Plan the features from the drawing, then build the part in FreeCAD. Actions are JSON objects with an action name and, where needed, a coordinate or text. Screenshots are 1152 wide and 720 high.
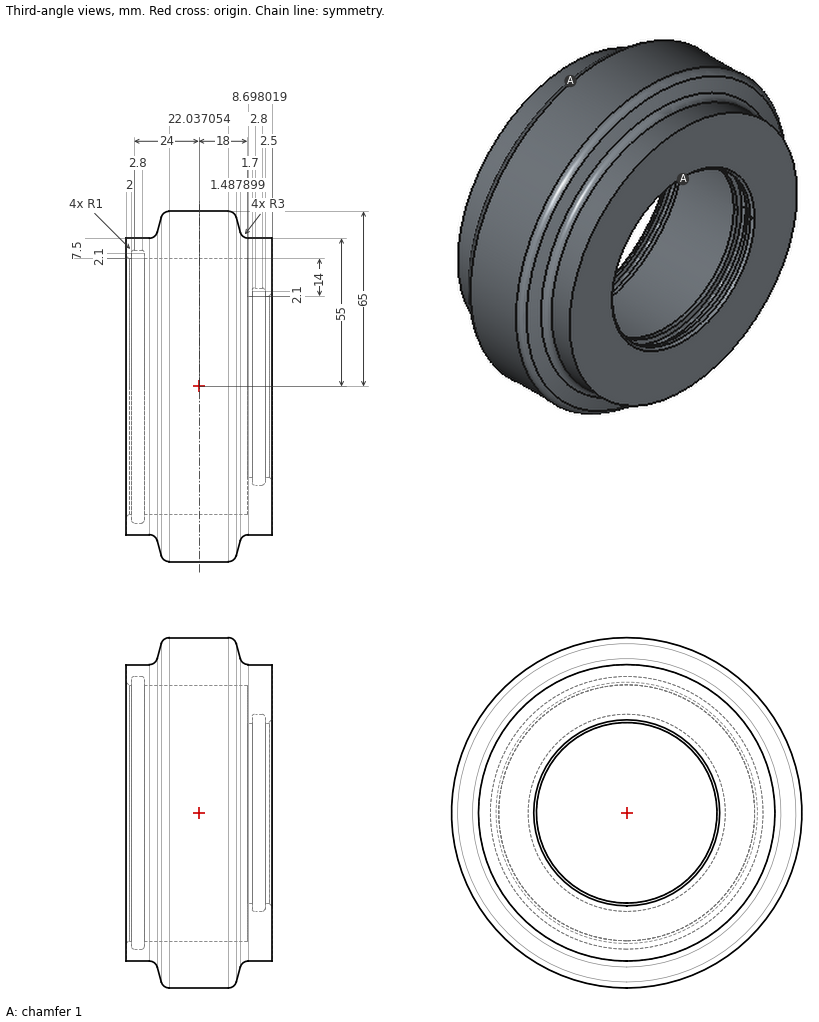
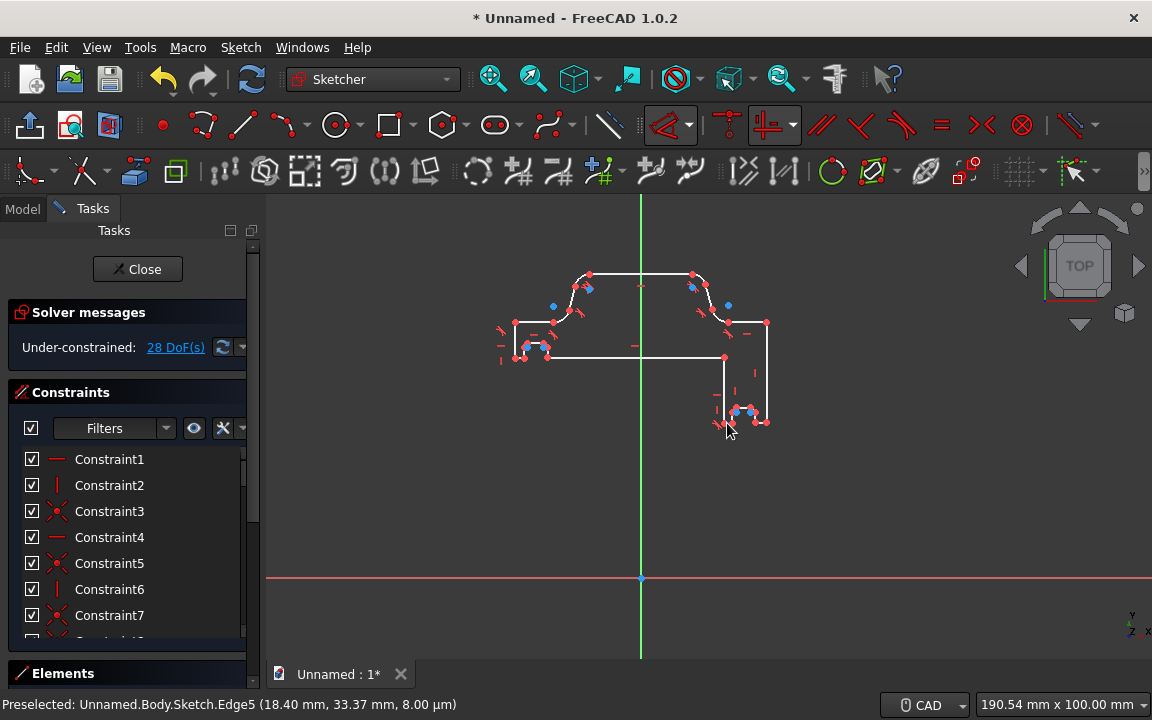
{"action": "scroll", "coordinate": [547, 346], "scroll_direction": "up", "scroll_amount": 10}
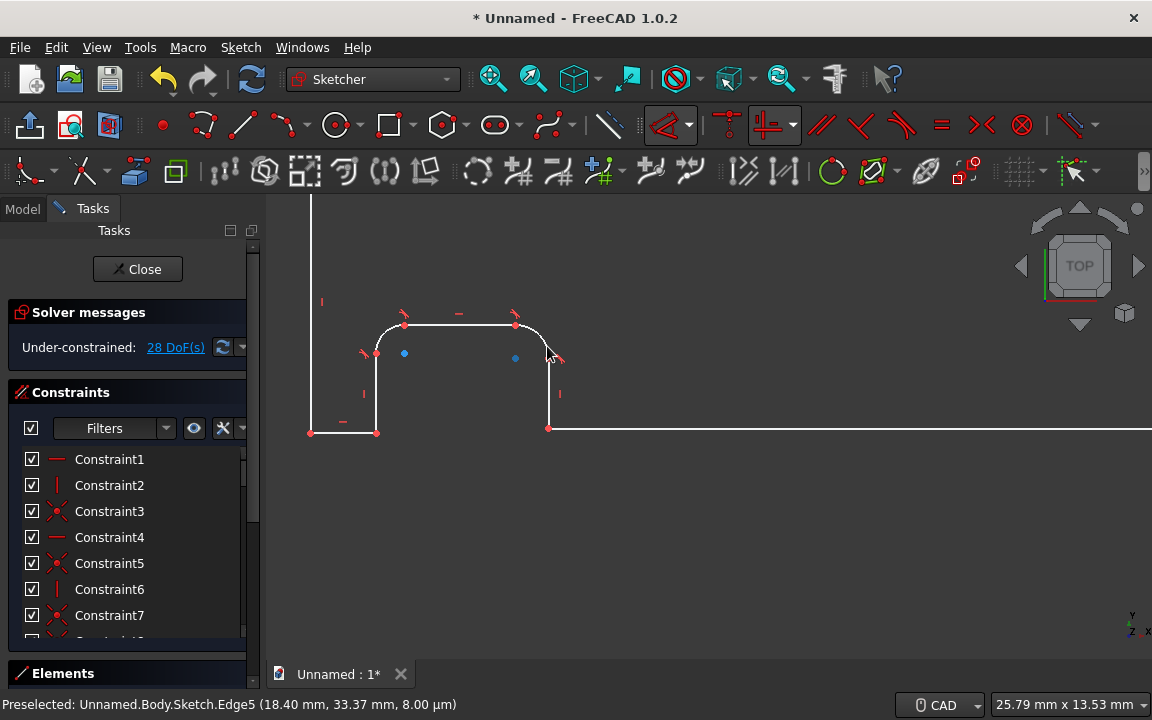
{"action": "left_click", "coordinate": [545, 343]}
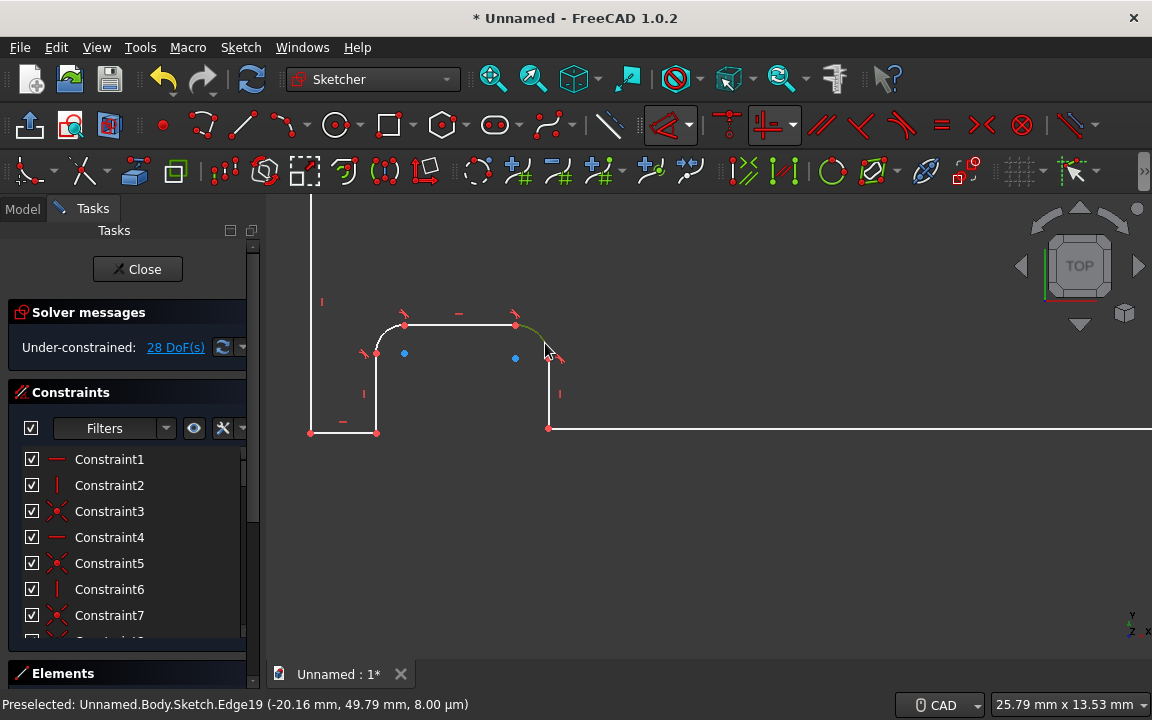
{"action": "scroll", "coordinate": [547, 346], "scroll_direction": "down", "scroll_amount": 10}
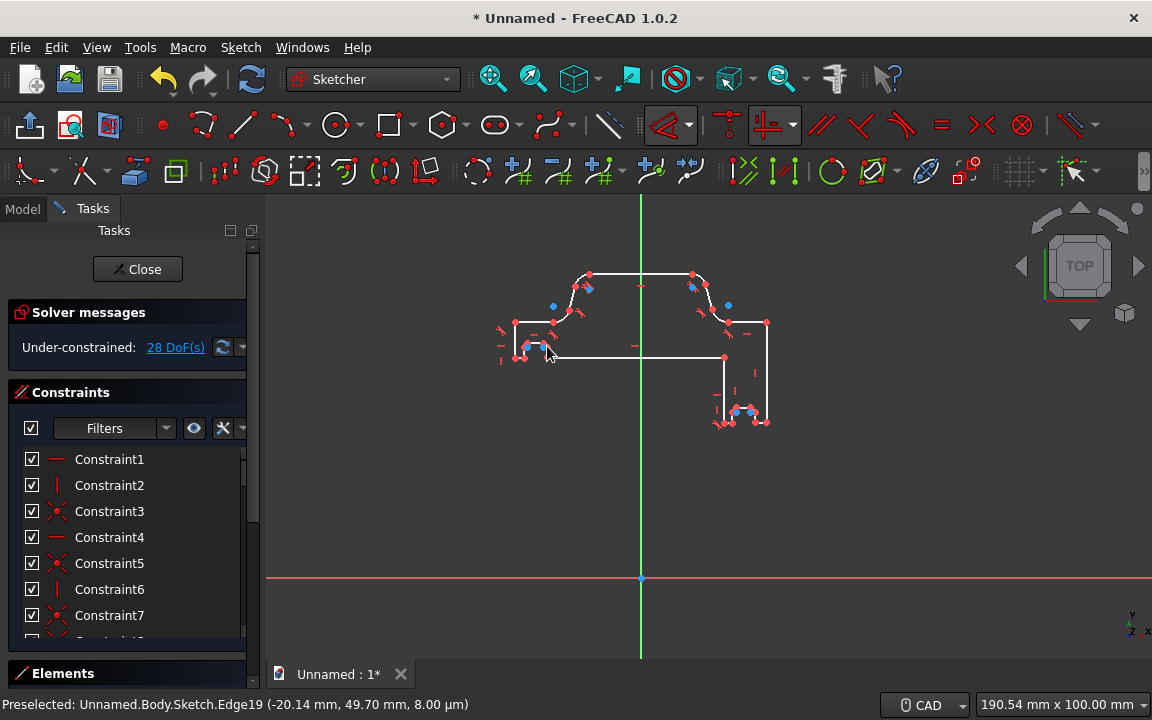
{"action": "scroll", "coordinate": [735, 408], "scroll_direction": "up", "scroll_amount": 10}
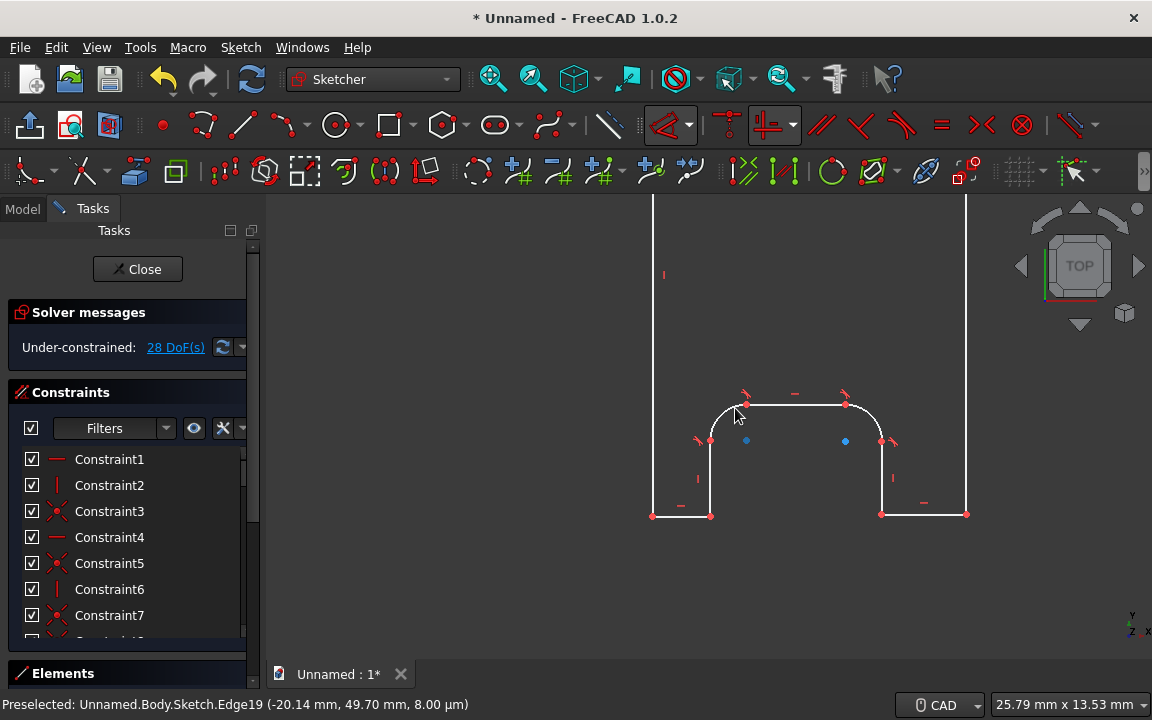
{"action": "left_click", "coordinate": [730, 409]}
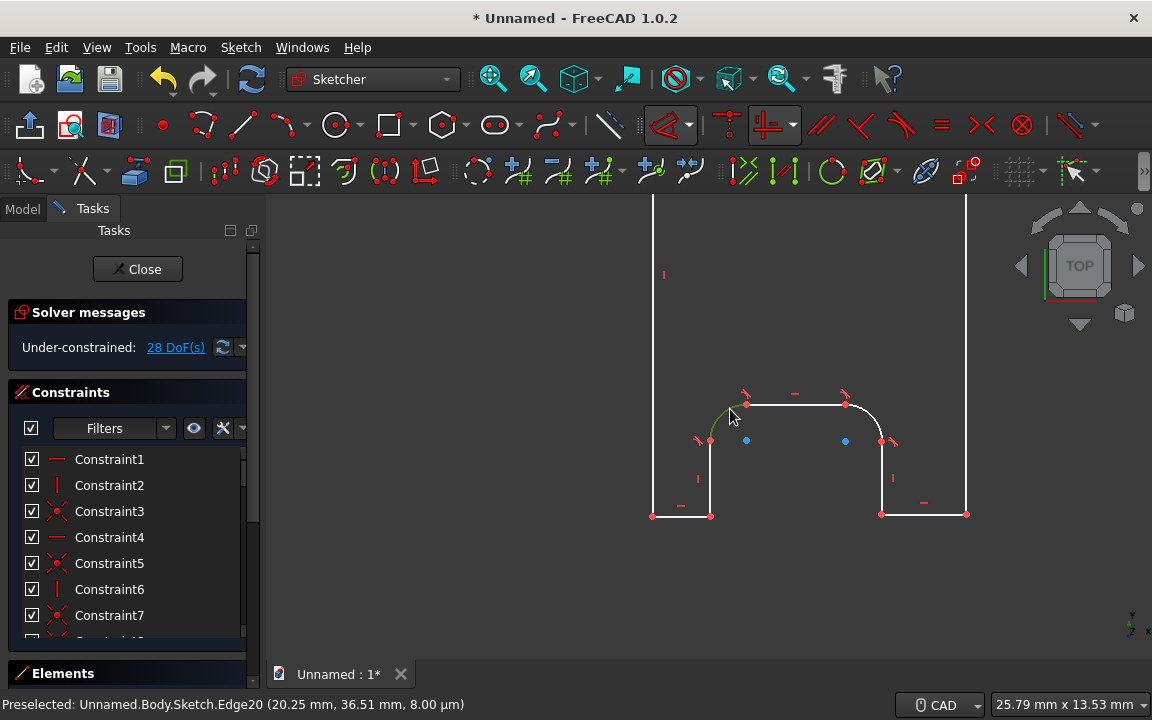
{"action": "left_click", "coordinate": [878, 425]}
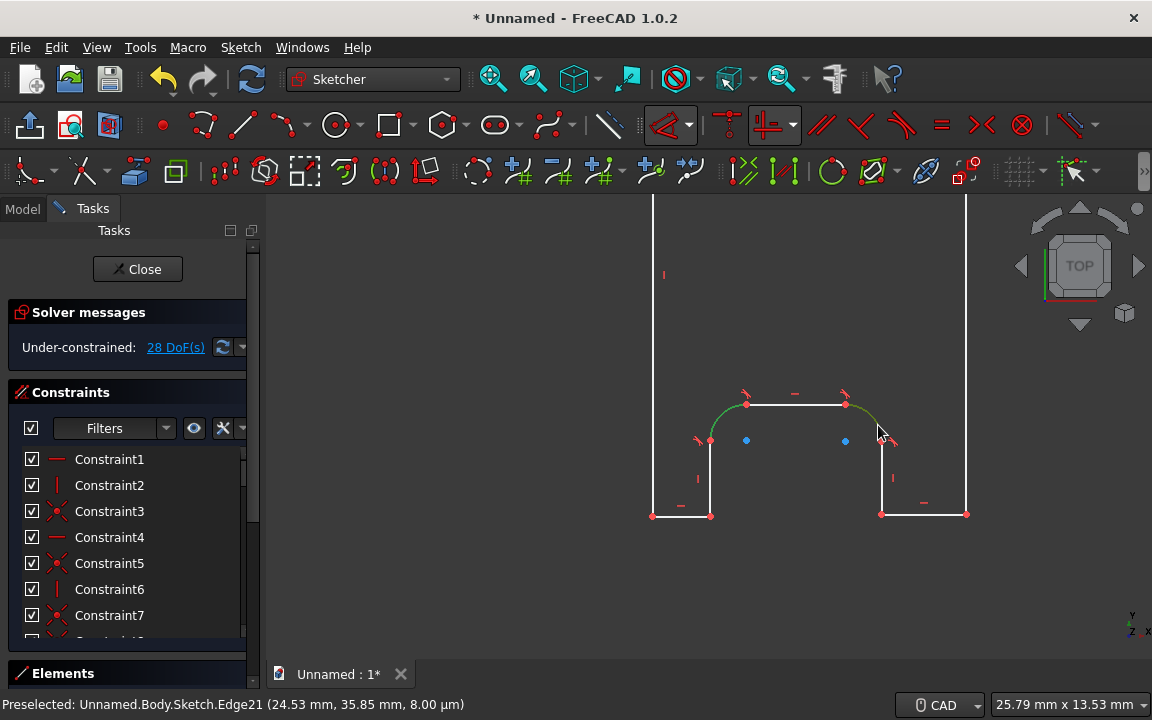
{"action": "scroll", "coordinate": [735, 408], "scroll_direction": "down", "scroll_amount": 10}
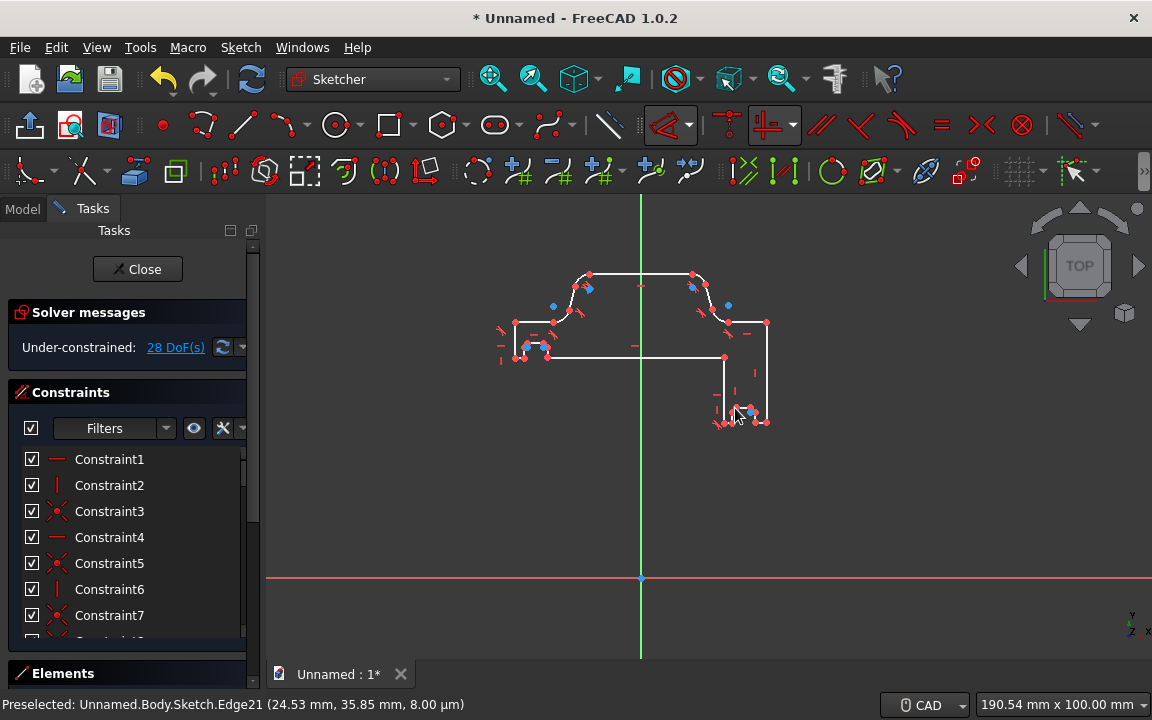
{"action": "scroll", "coordinate": [526, 344], "scroll_direction": "up", "scroll_amount": 11}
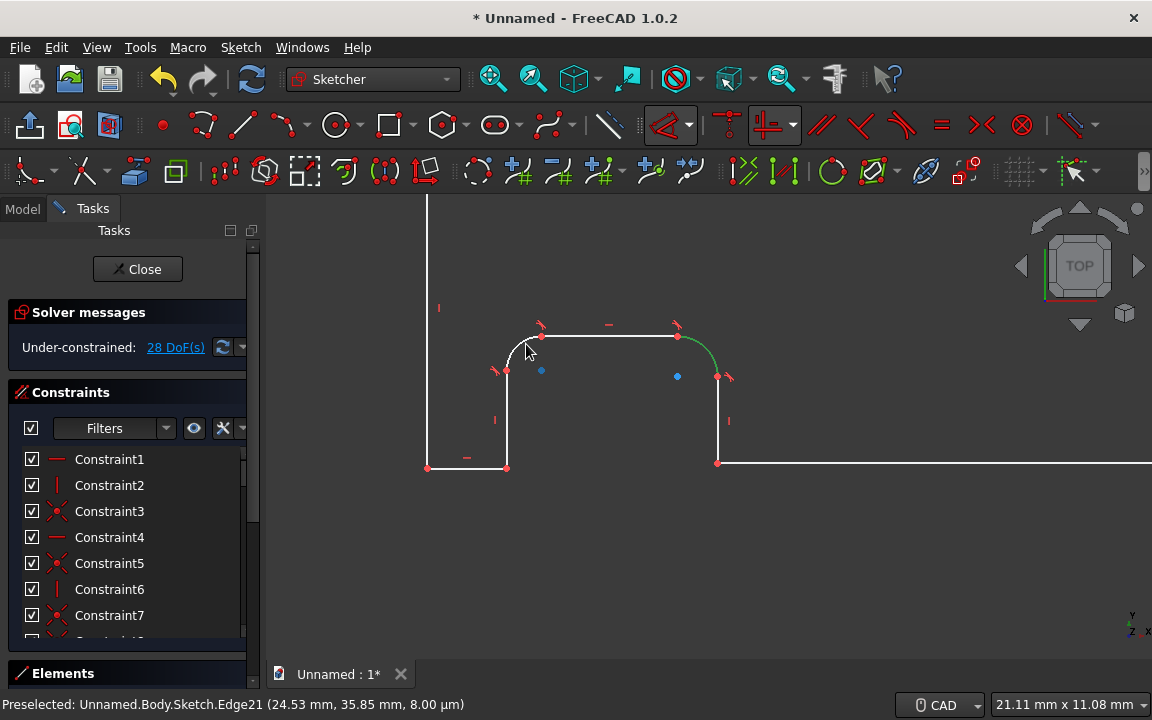
{"action": "left_click", "coordinate": [526, 340]}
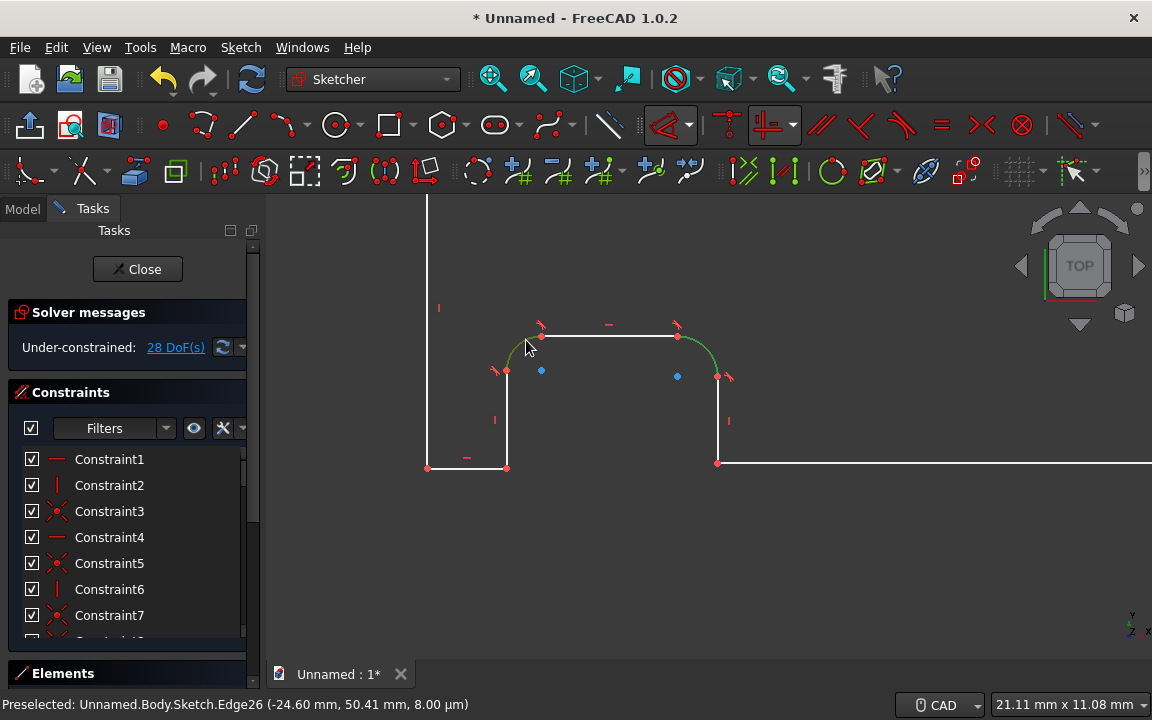
{"action": "left_click", "coordinate": [942, 126]}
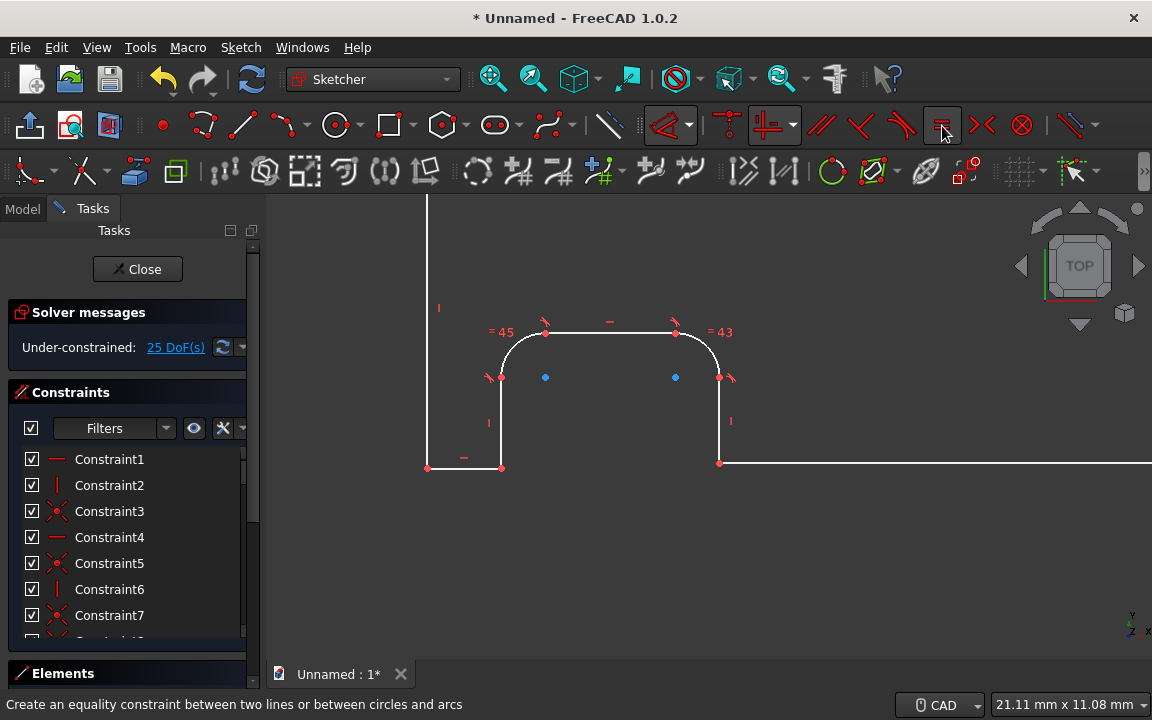
{"action": "scroll", "coordinate": [526, 344], "scroll_direction": "down", "scroll_amount": 11}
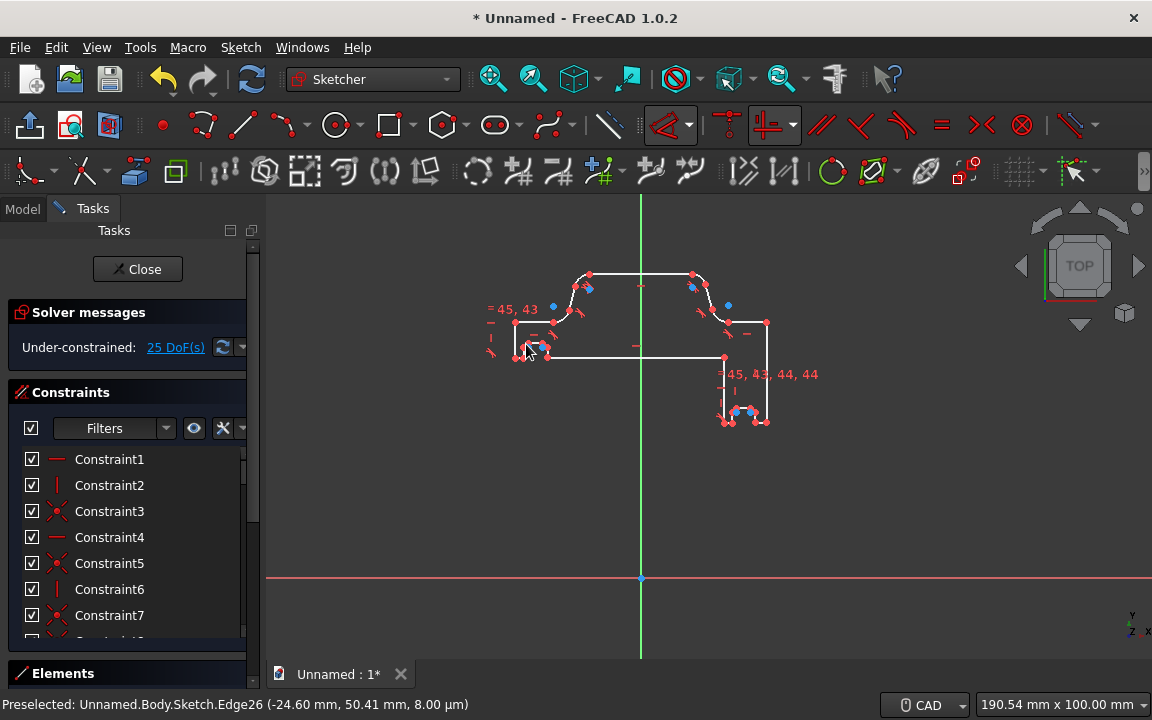
{"action": "scroll", "coordinate": [715, 316], "scroll_direction": "up", "scroll_amount": 4}